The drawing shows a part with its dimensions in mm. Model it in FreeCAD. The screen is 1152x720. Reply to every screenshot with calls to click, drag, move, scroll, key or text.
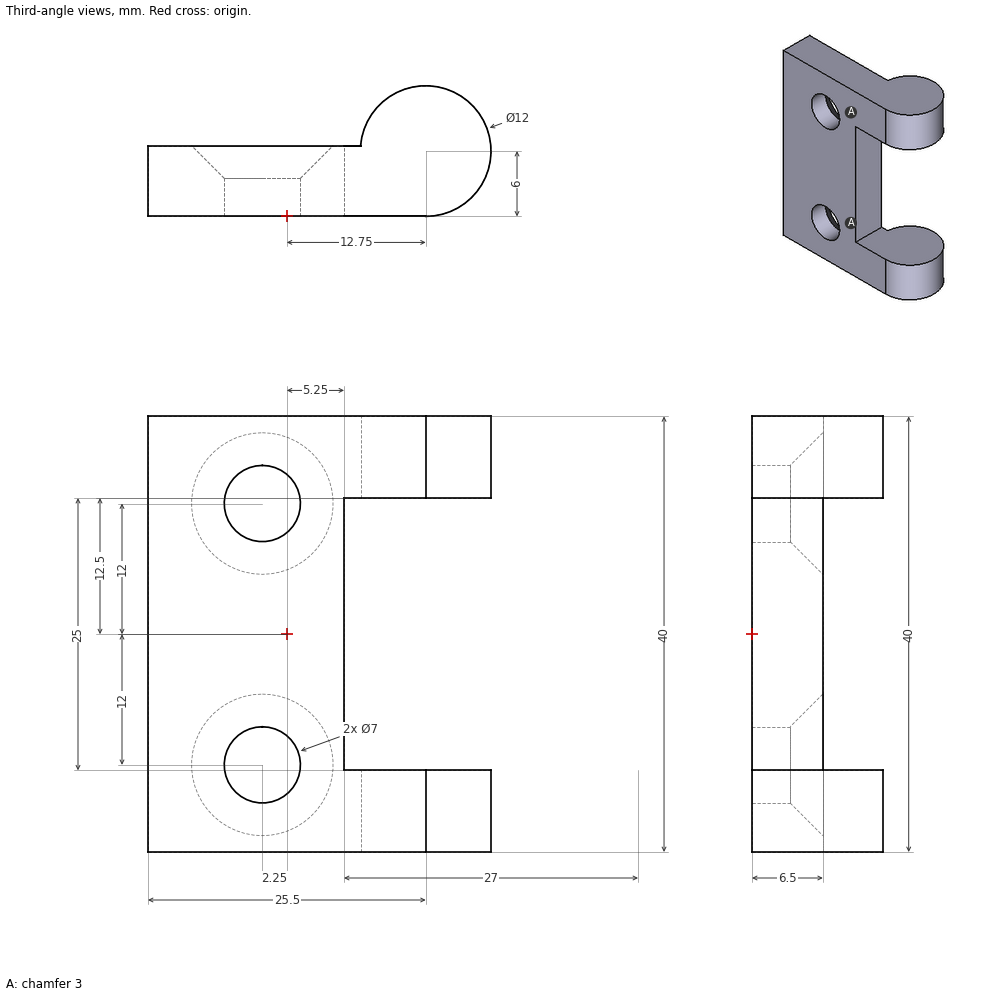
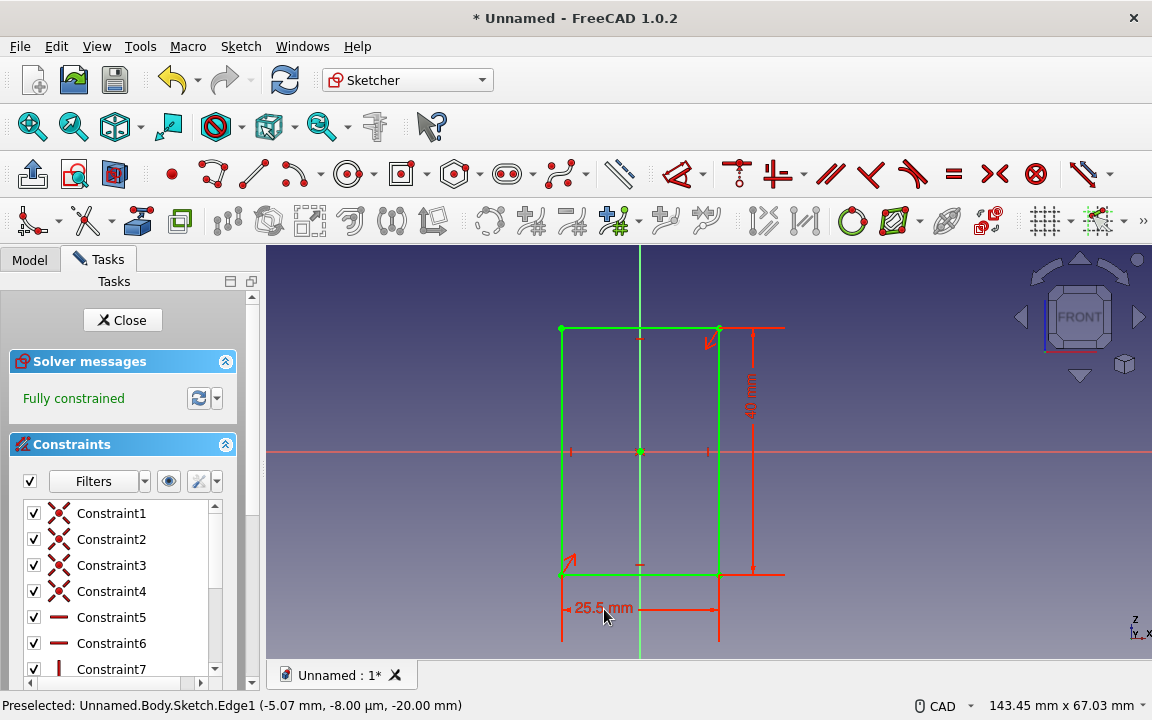
click(123, 320)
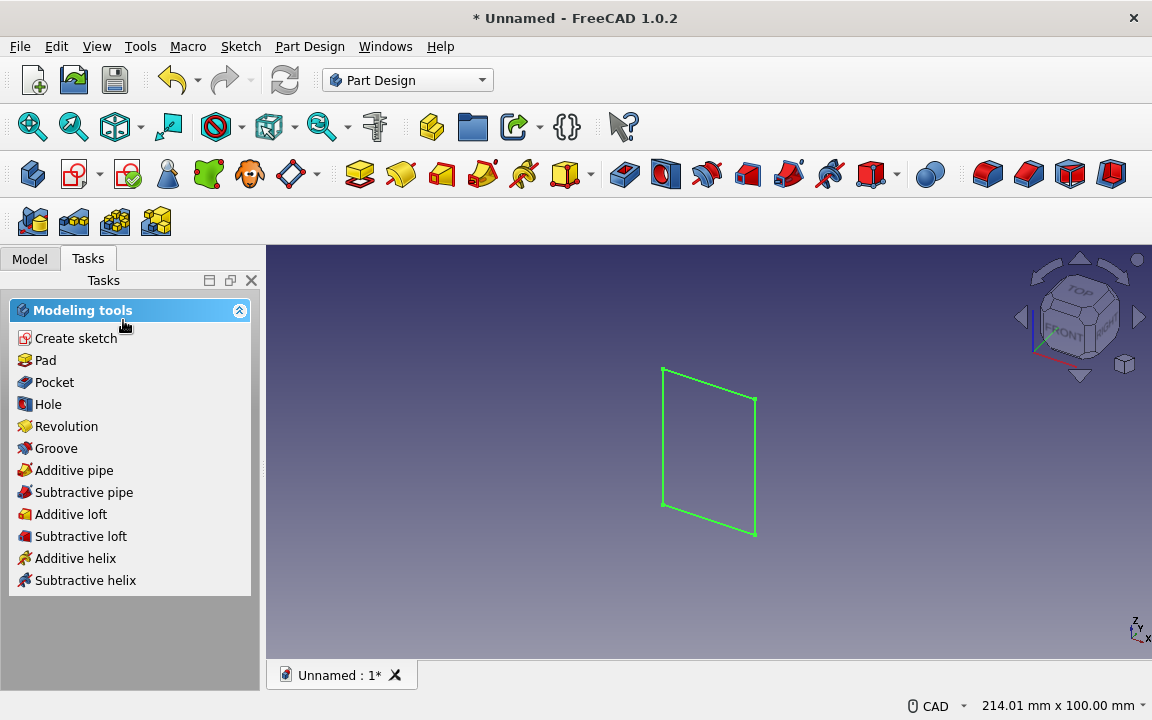
click(360, 174)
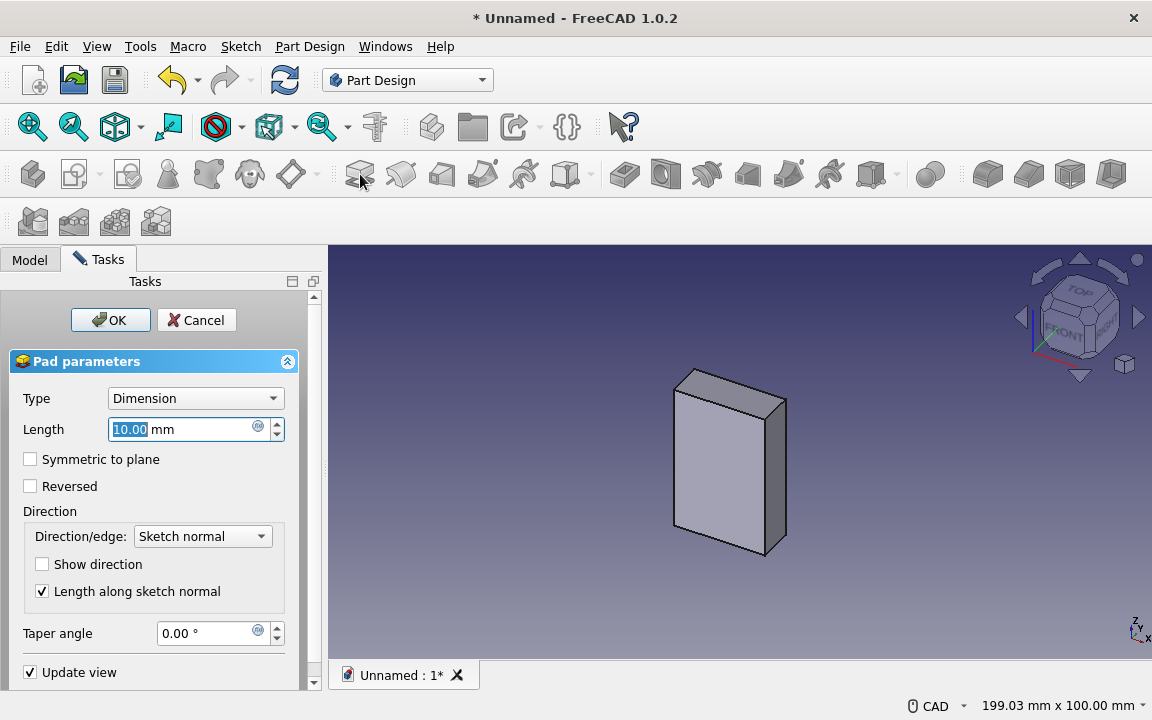
text(6.5)
key(Tab)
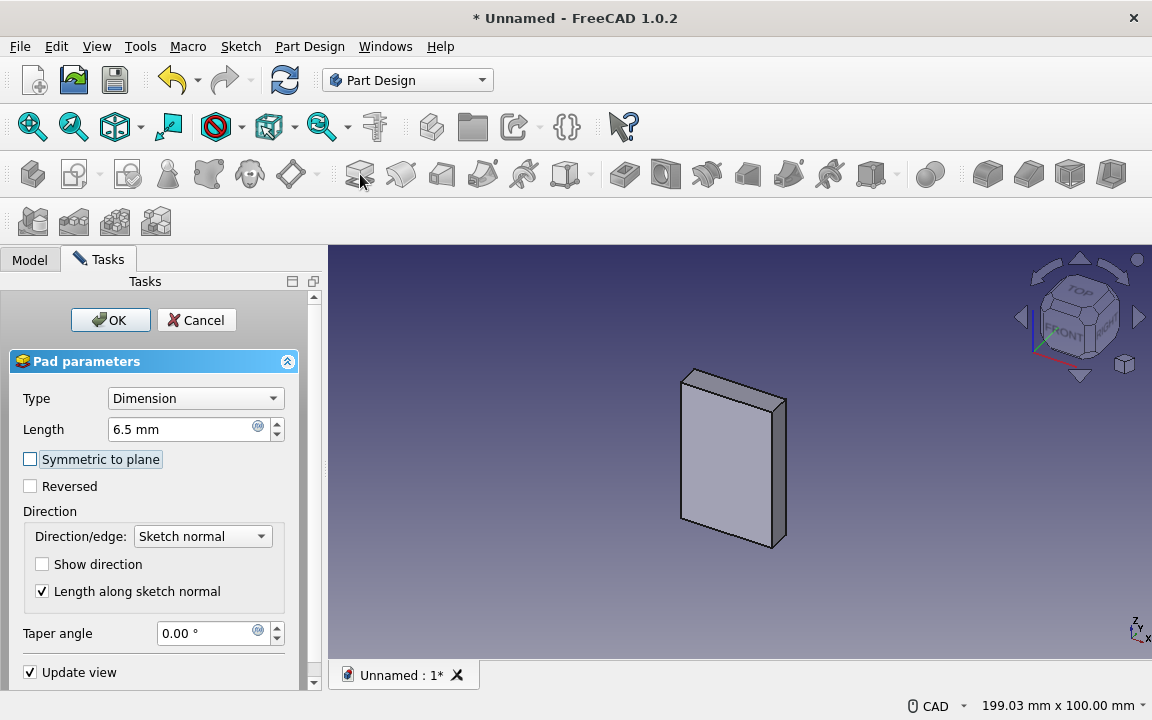
click(31, 486)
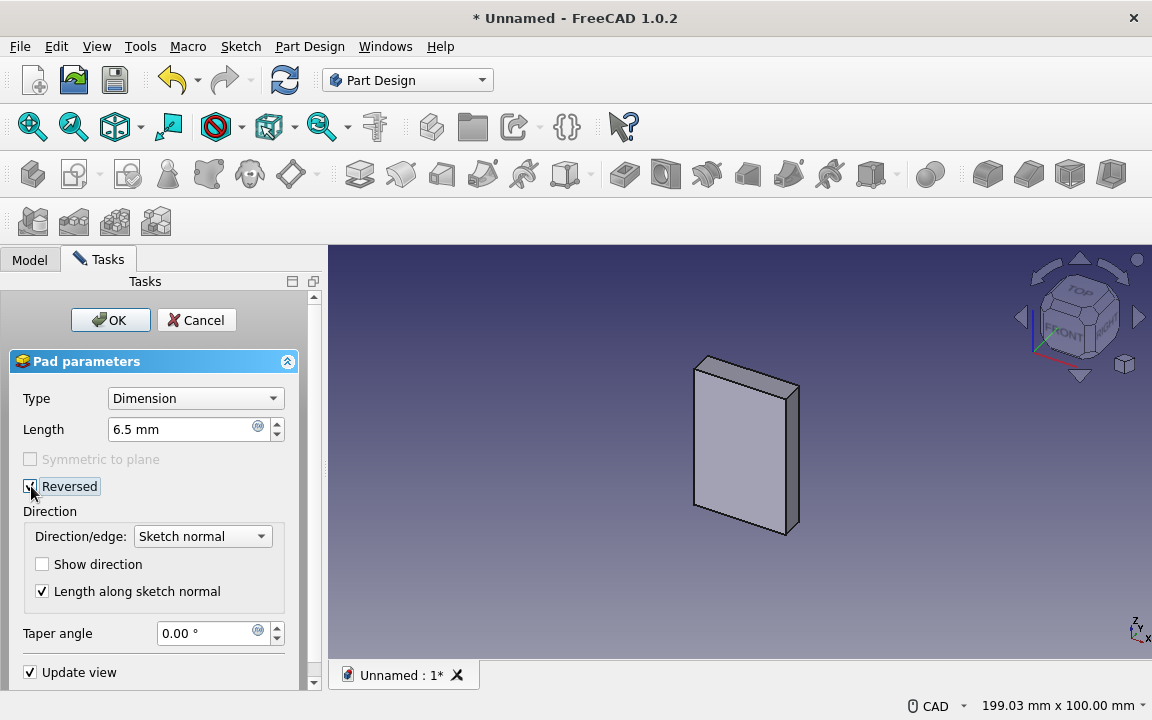
click(111, 320)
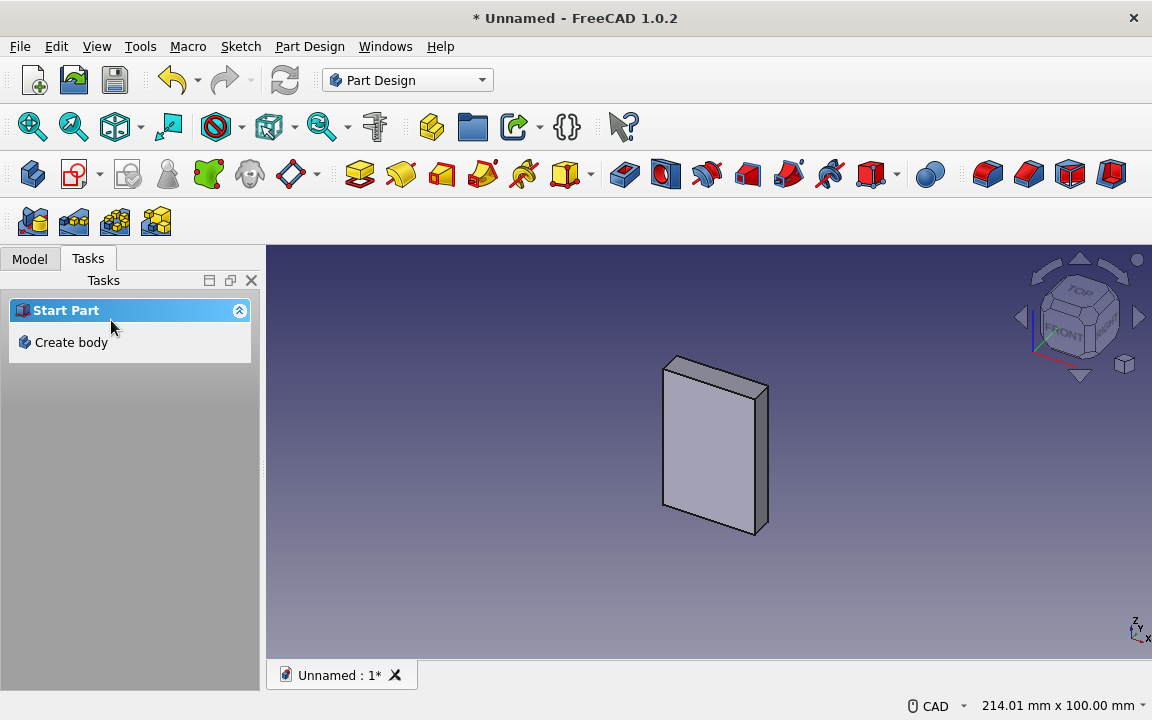
click(33, 128)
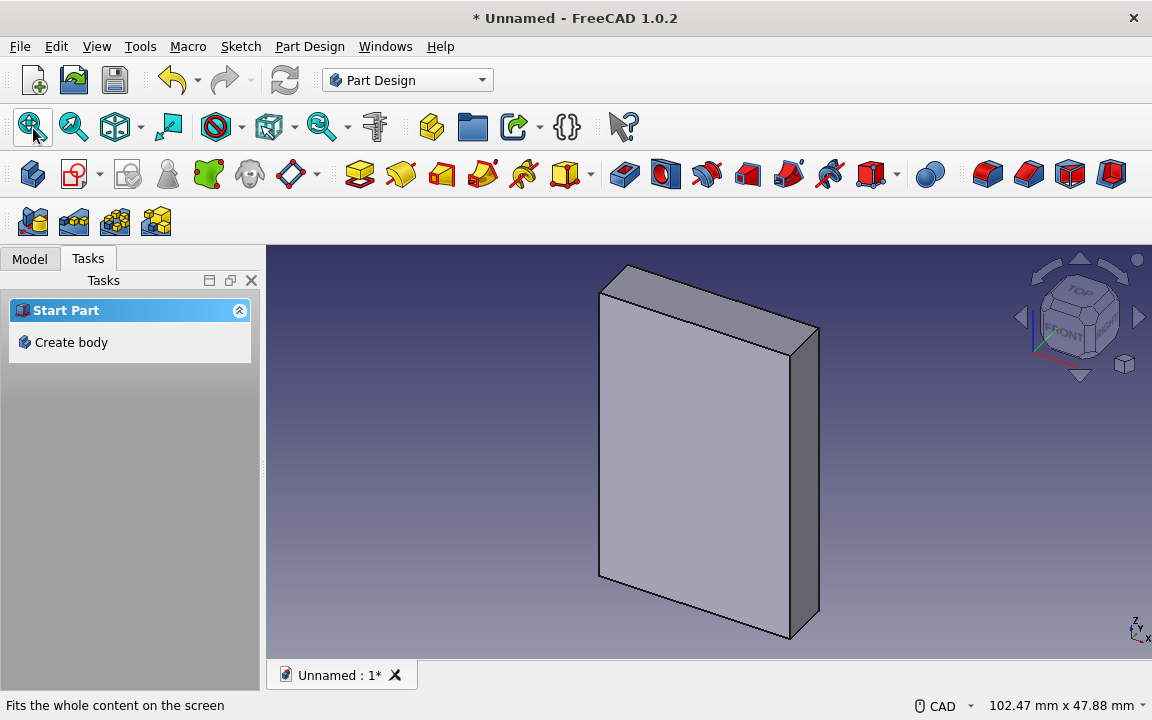
click(764, 327)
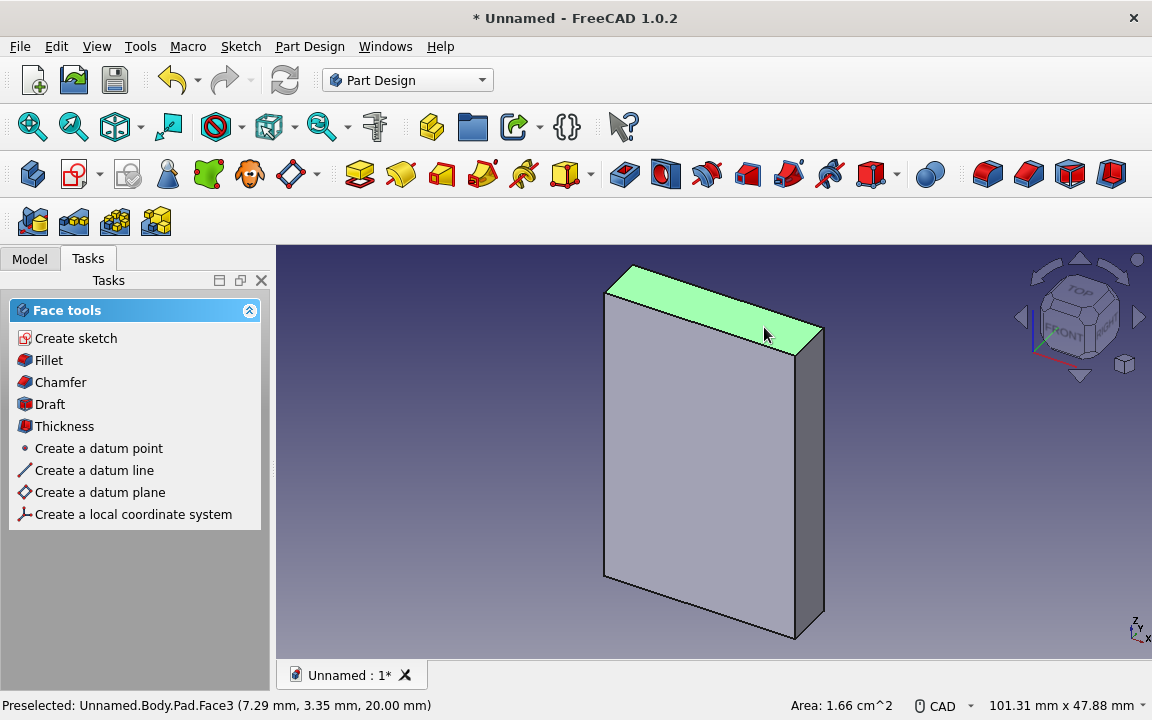
click(74, 174)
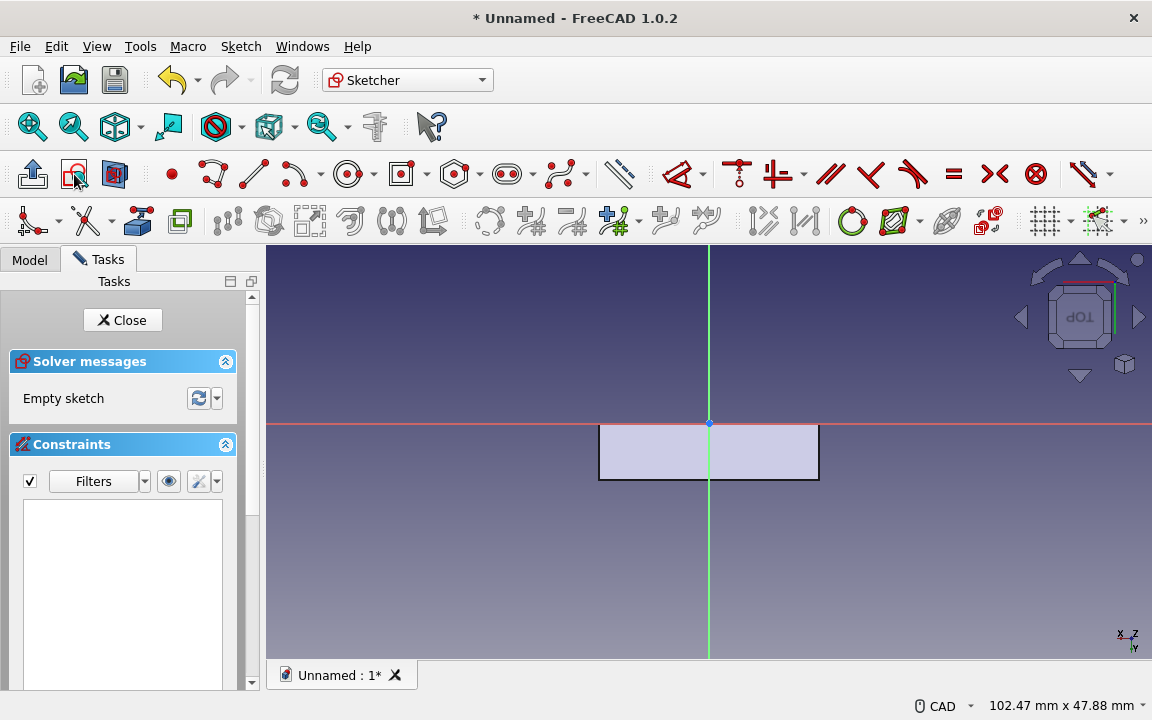
scroll(618, 495, up, 4)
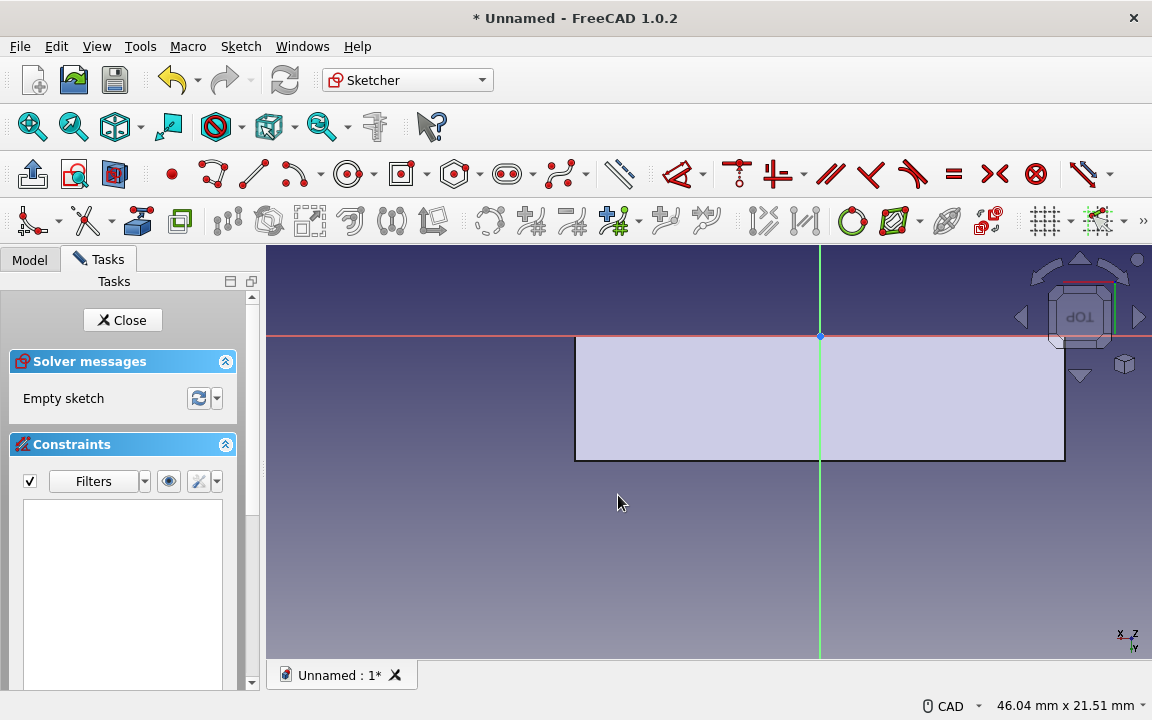
click(348, 174)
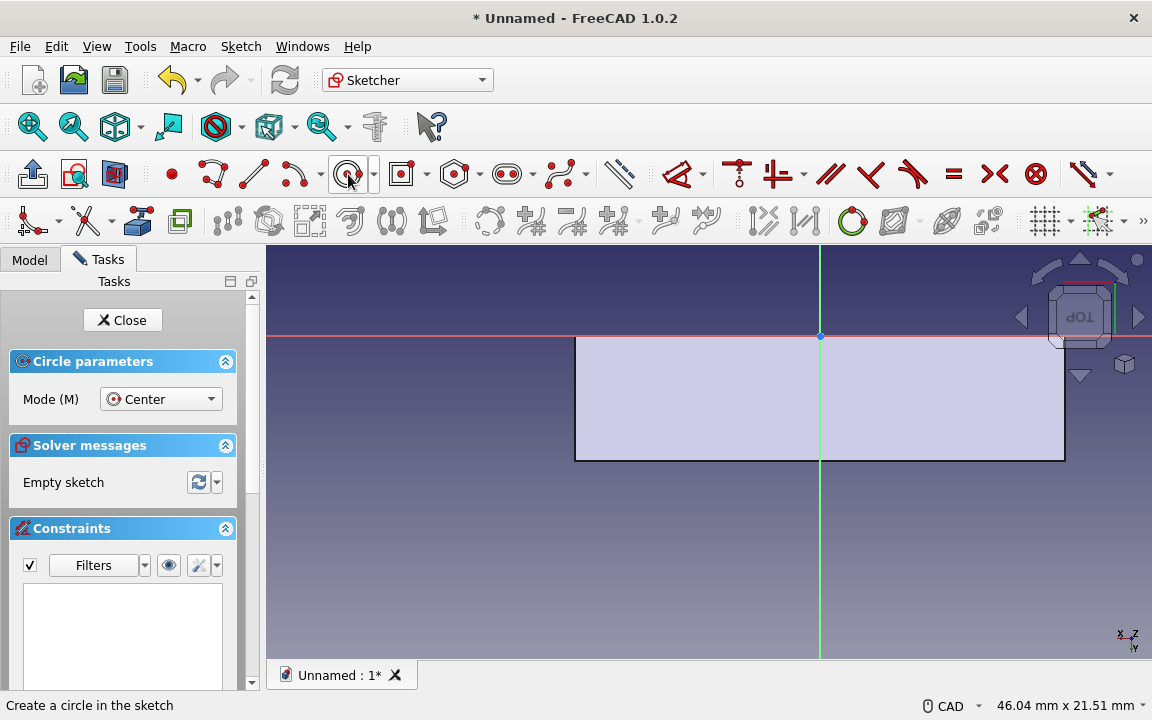
click(575, 451)
click(656, 370)
key(Escape)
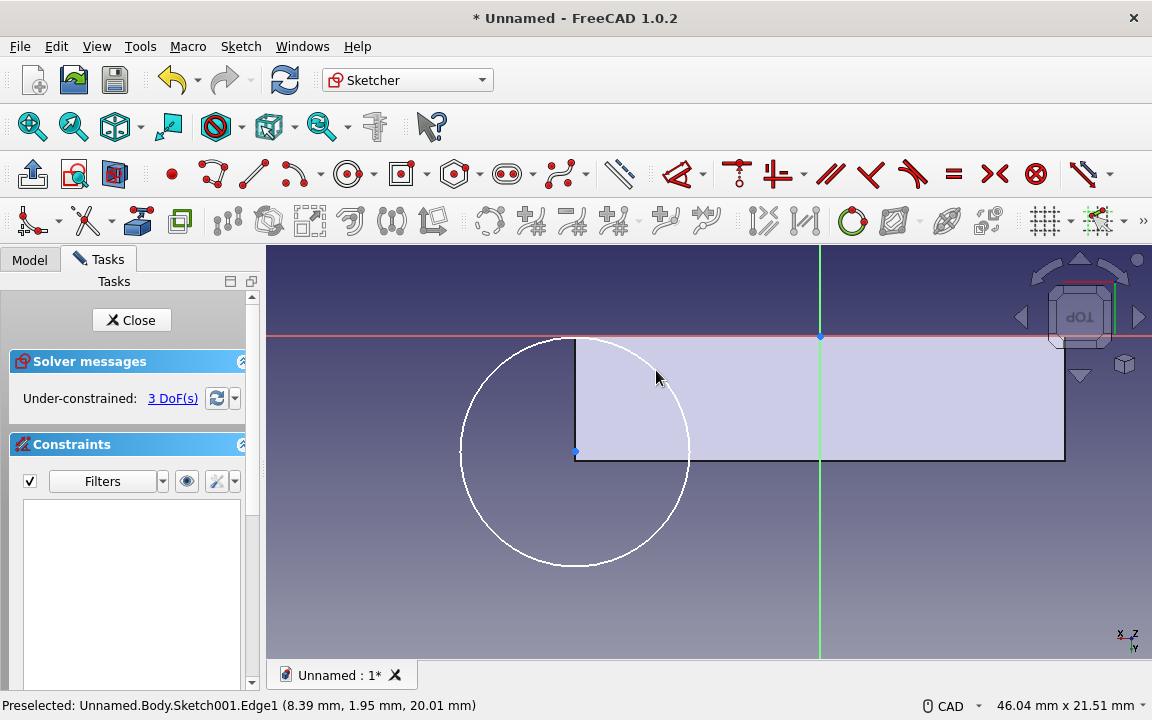
click(676, 174)